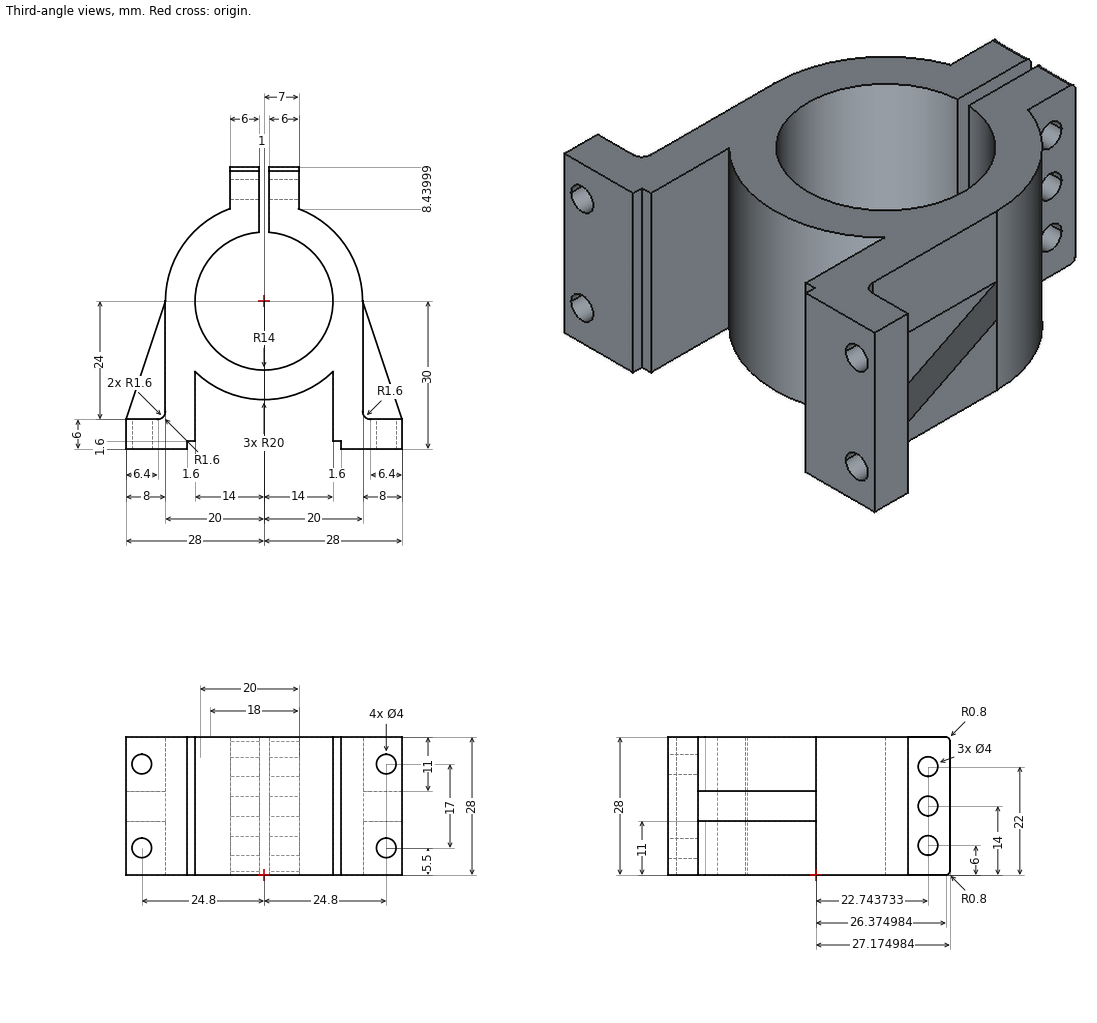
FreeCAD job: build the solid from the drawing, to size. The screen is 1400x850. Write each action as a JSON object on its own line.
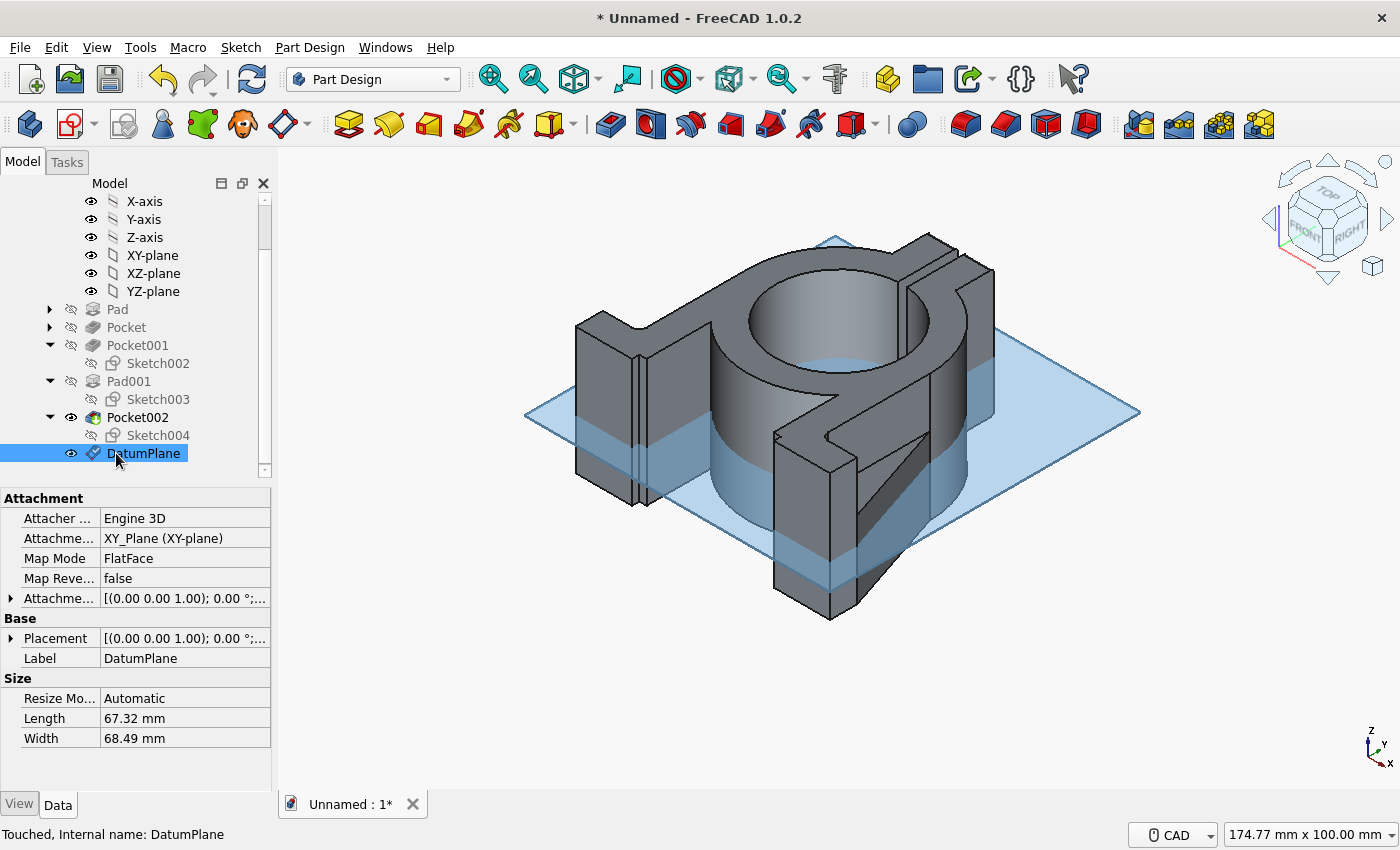
{"action": "left_click", "coordinate": [70, 124]}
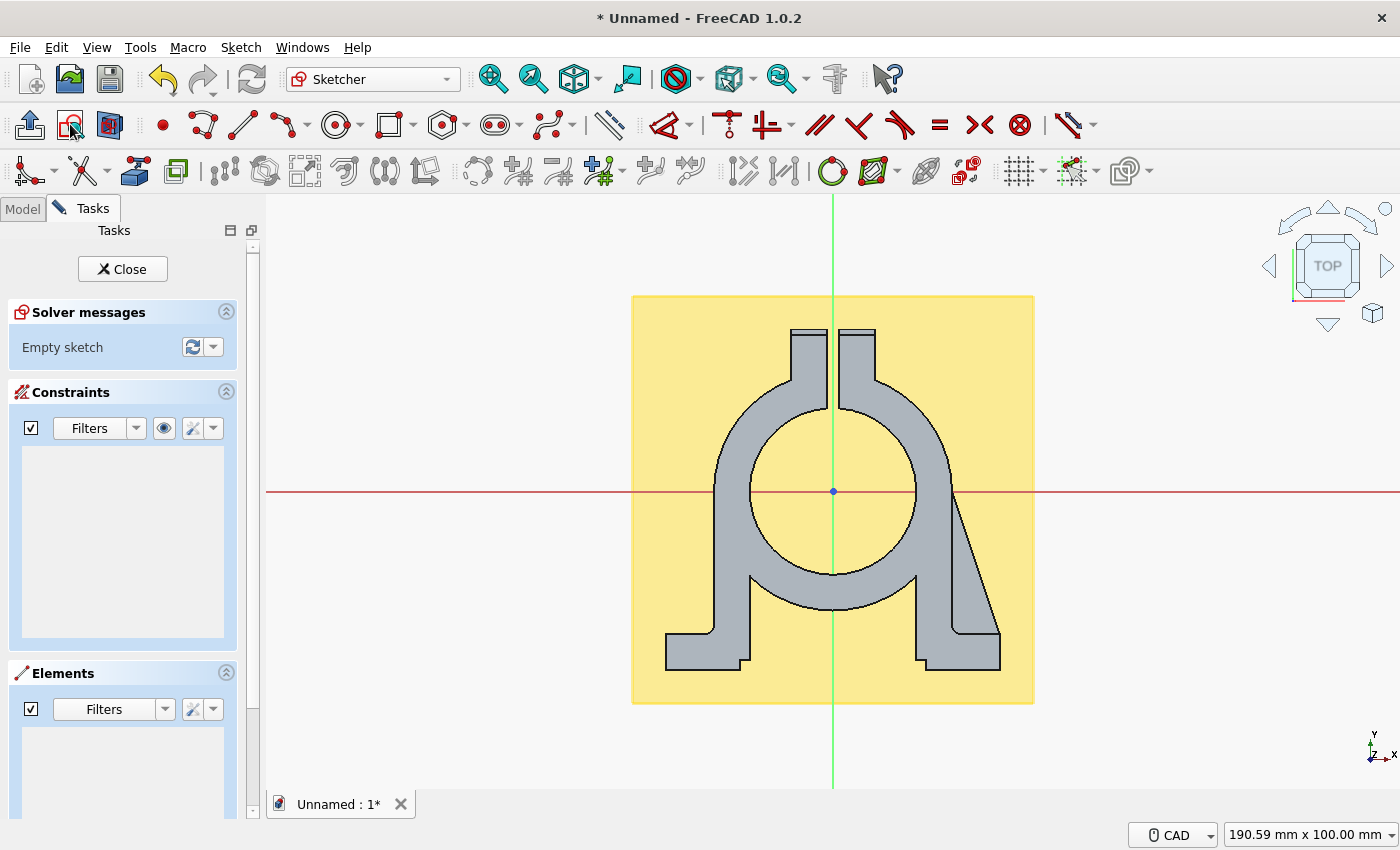
{"action": "left_click", "coordinate": [110, 126]}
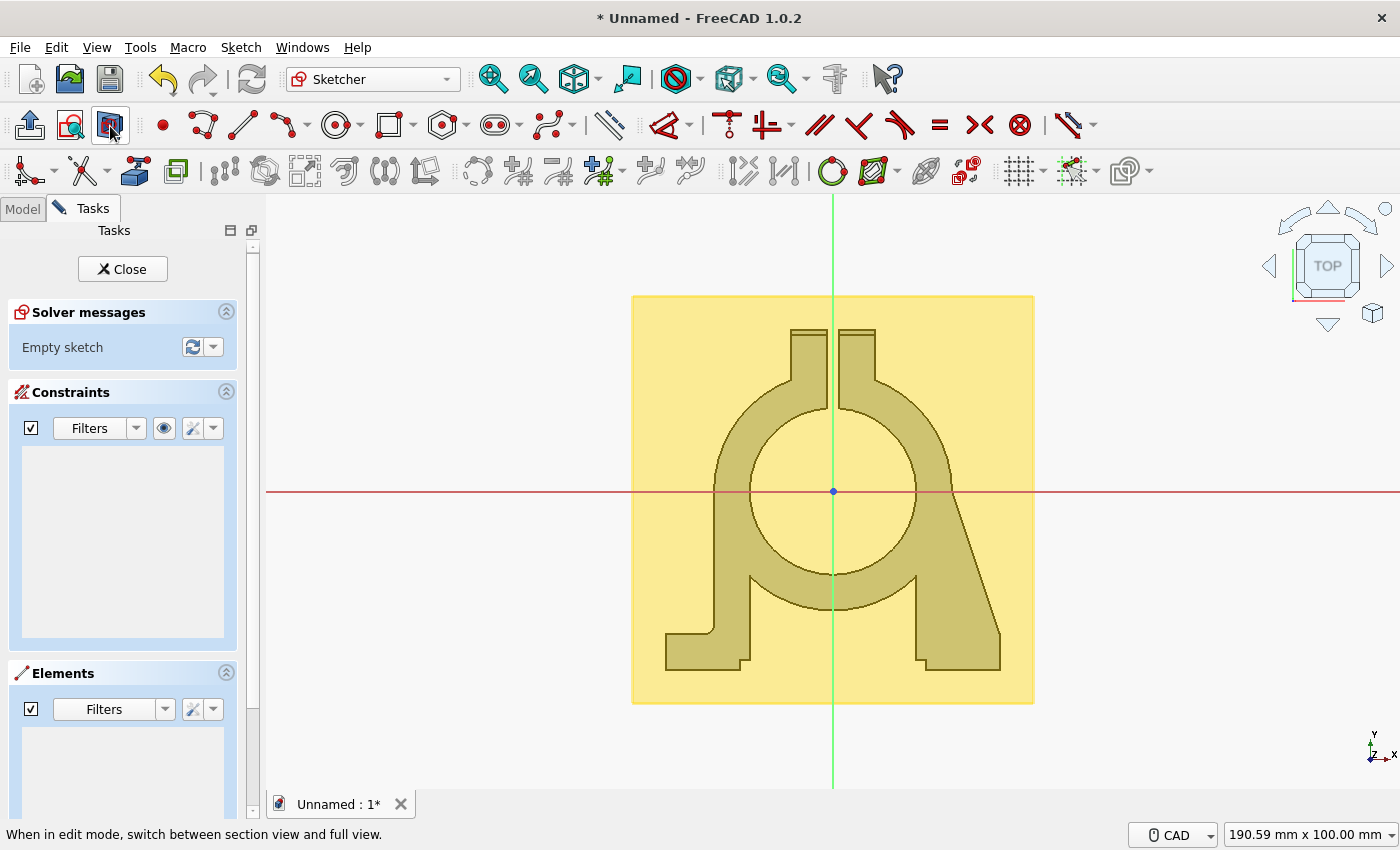
{"action": "scroll", "coordinate": [1005, 604], "scroll_direction": "up", "scroll_amount": 5}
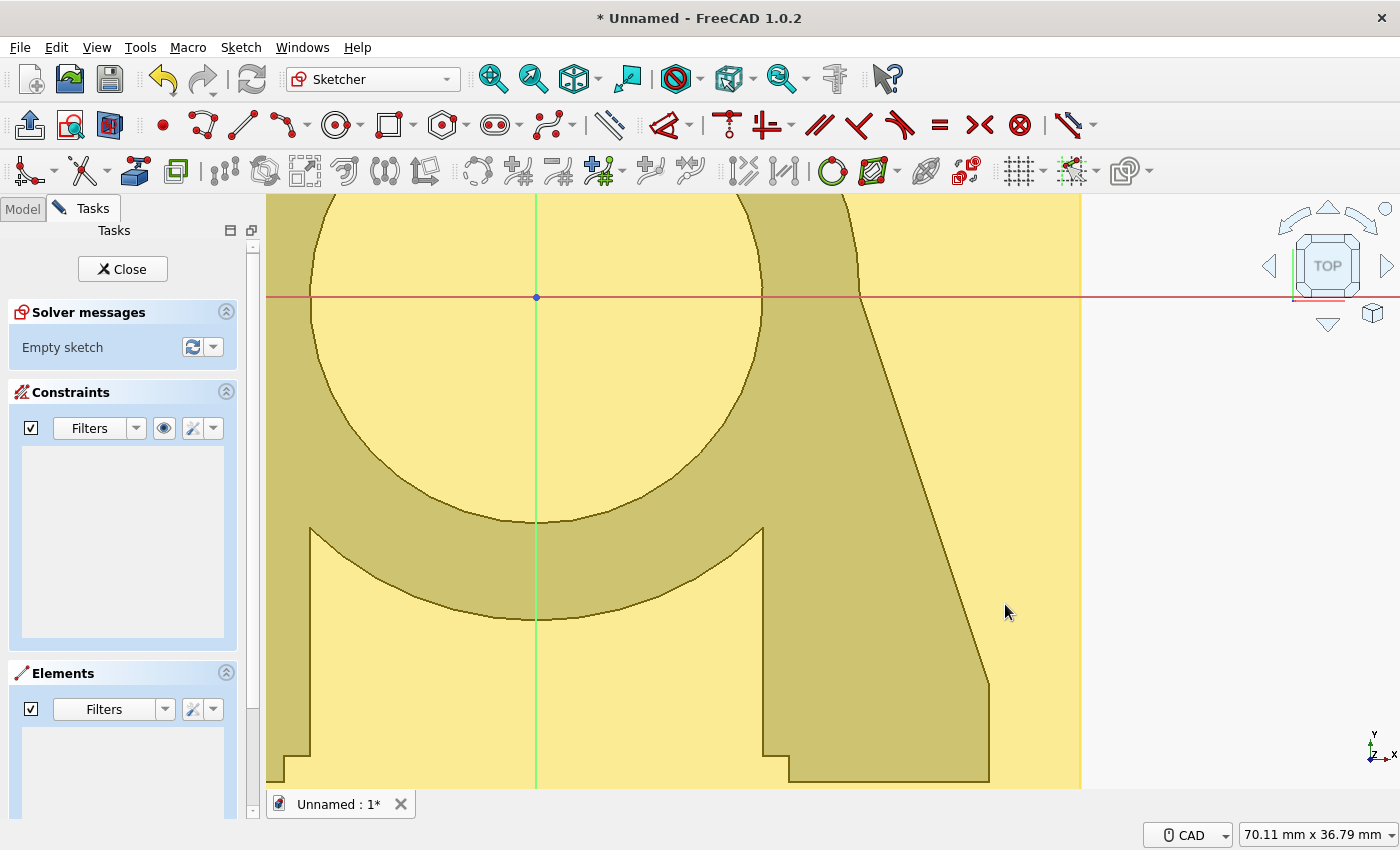
{"action": "left_click", "coordinate": [204, 126]}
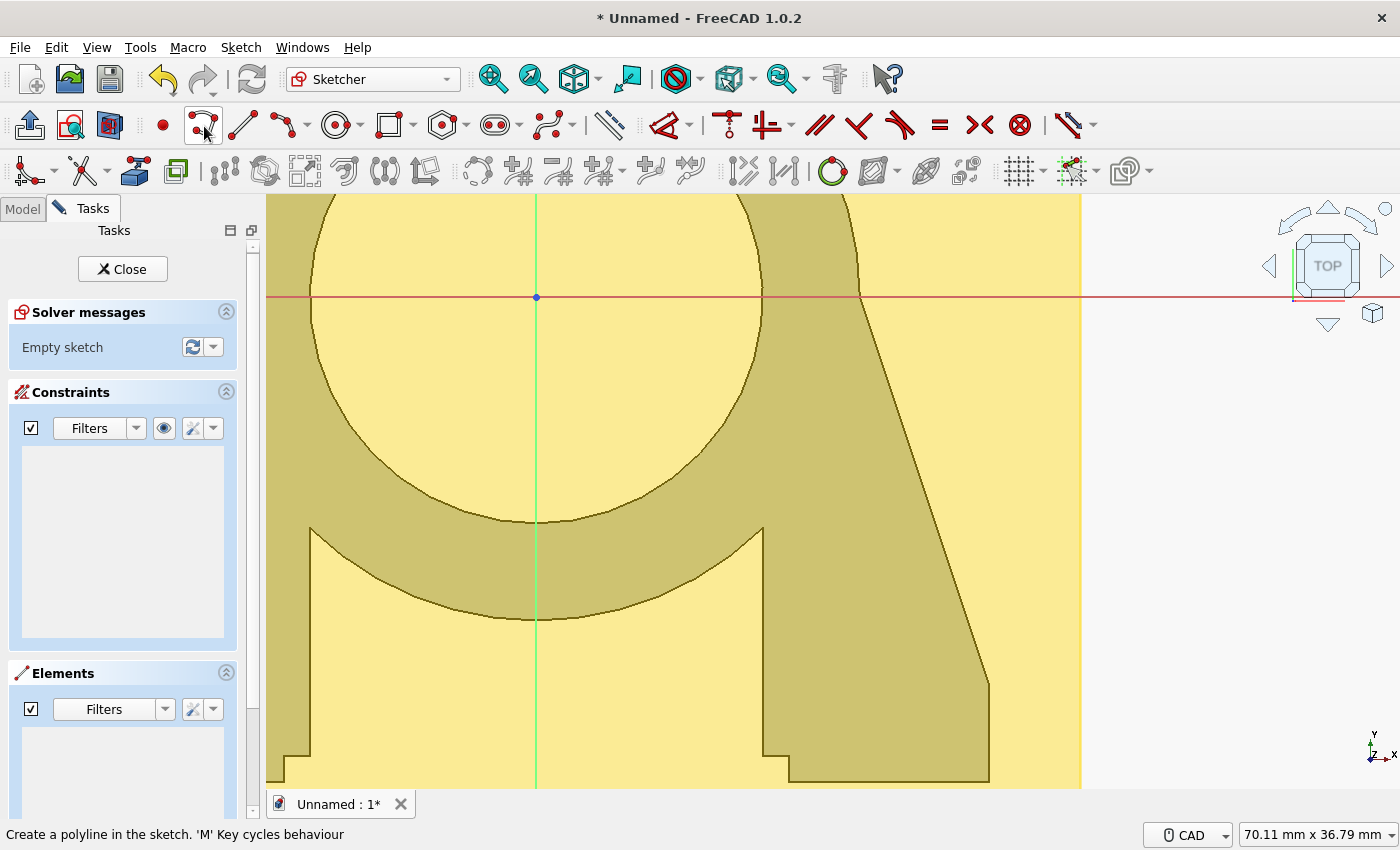
{"action": "left_click", "coordinate": [860, 659]}
{"action": "left_click", "coordinate": [860, 297]}
{"action": "left_click", "coordinate": [989, 685]}
{"action": "left_click", "coordinate": [886, 685]}
{"action": "right_click", "coordinate": [886, 685]}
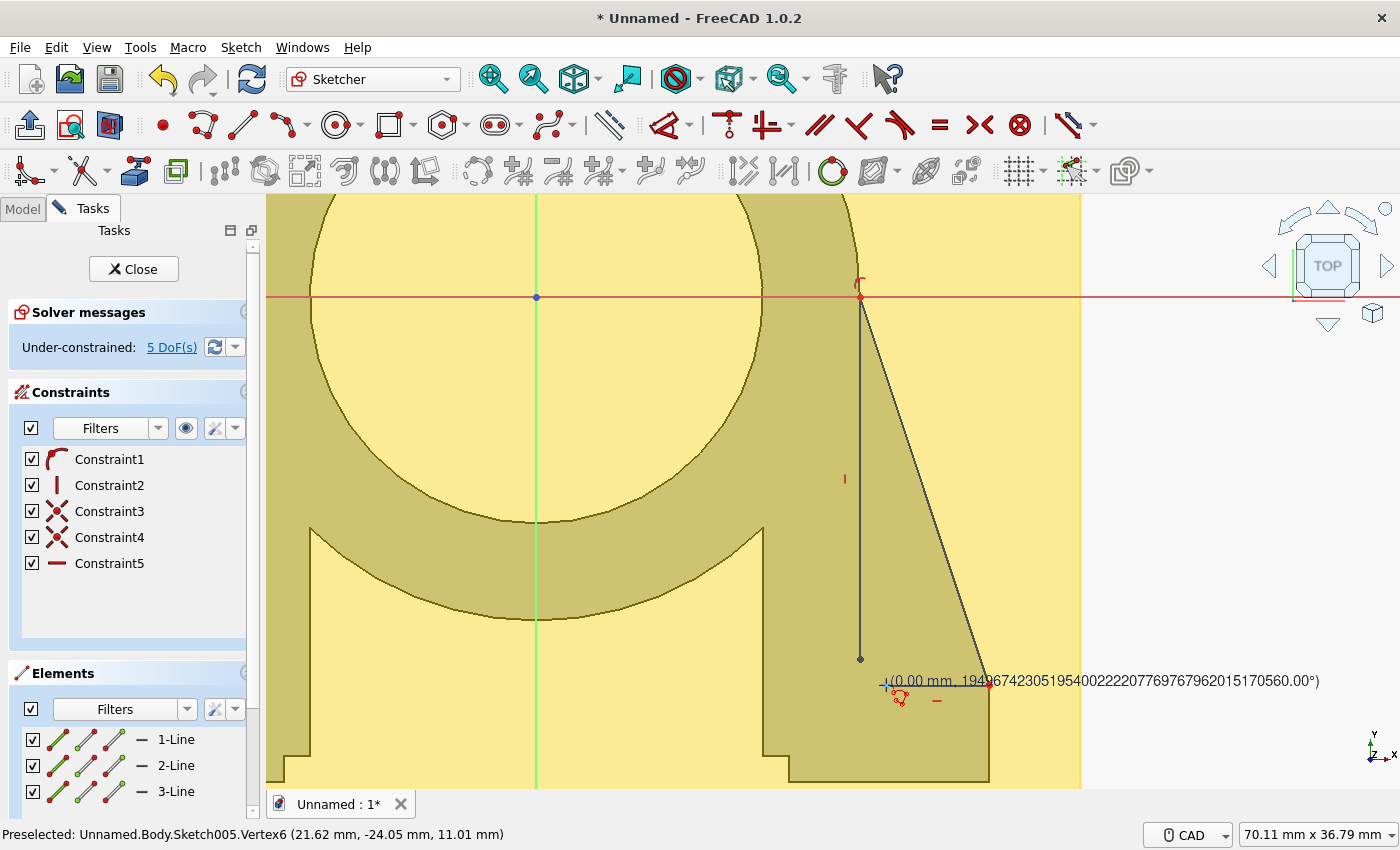
{"action": "left_click", "coordinate": [284, 126]}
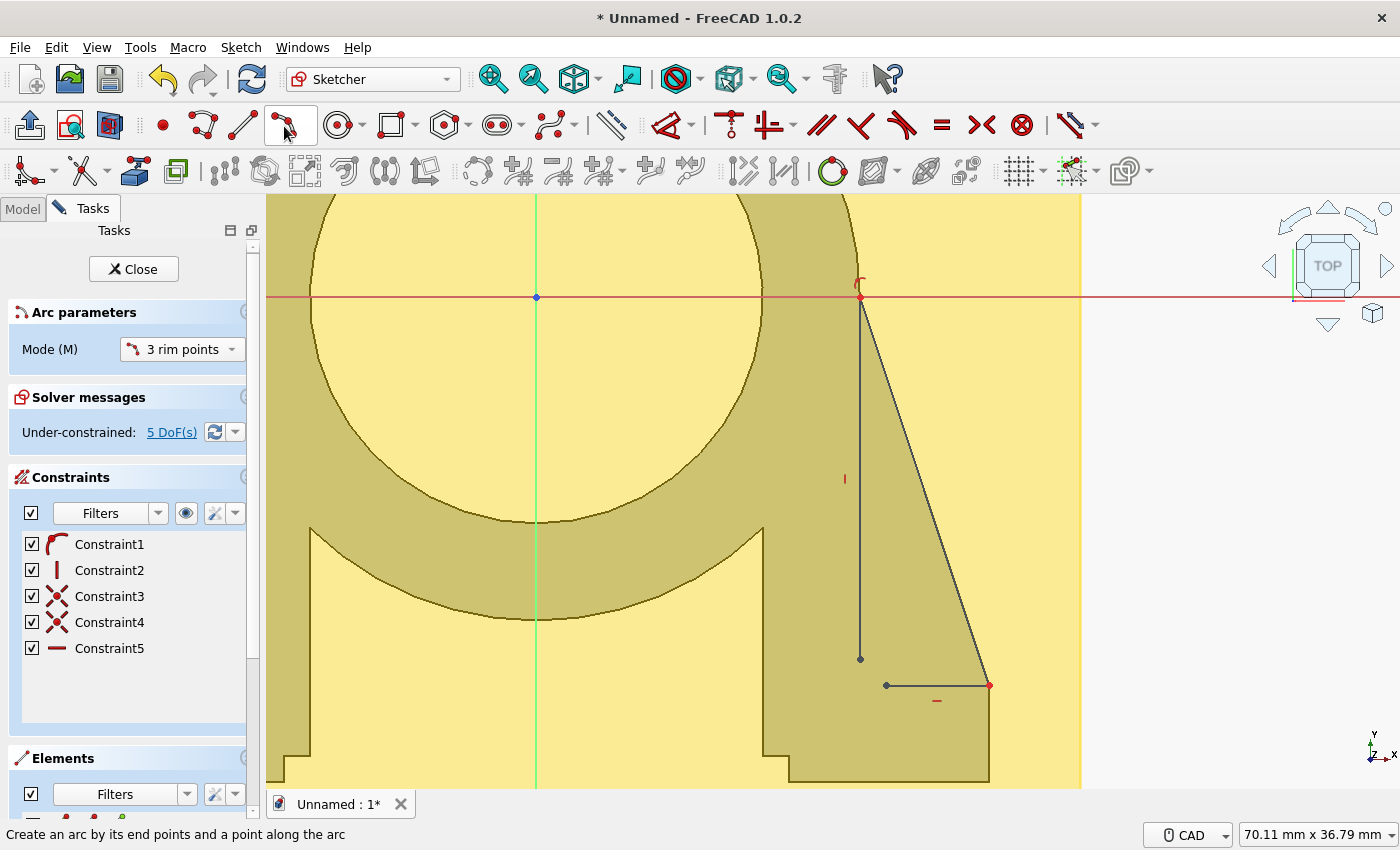
{"action": "left_click", "coordinate": [886, 686]}
{"action": "left_click", "coordinate": [860, 660]}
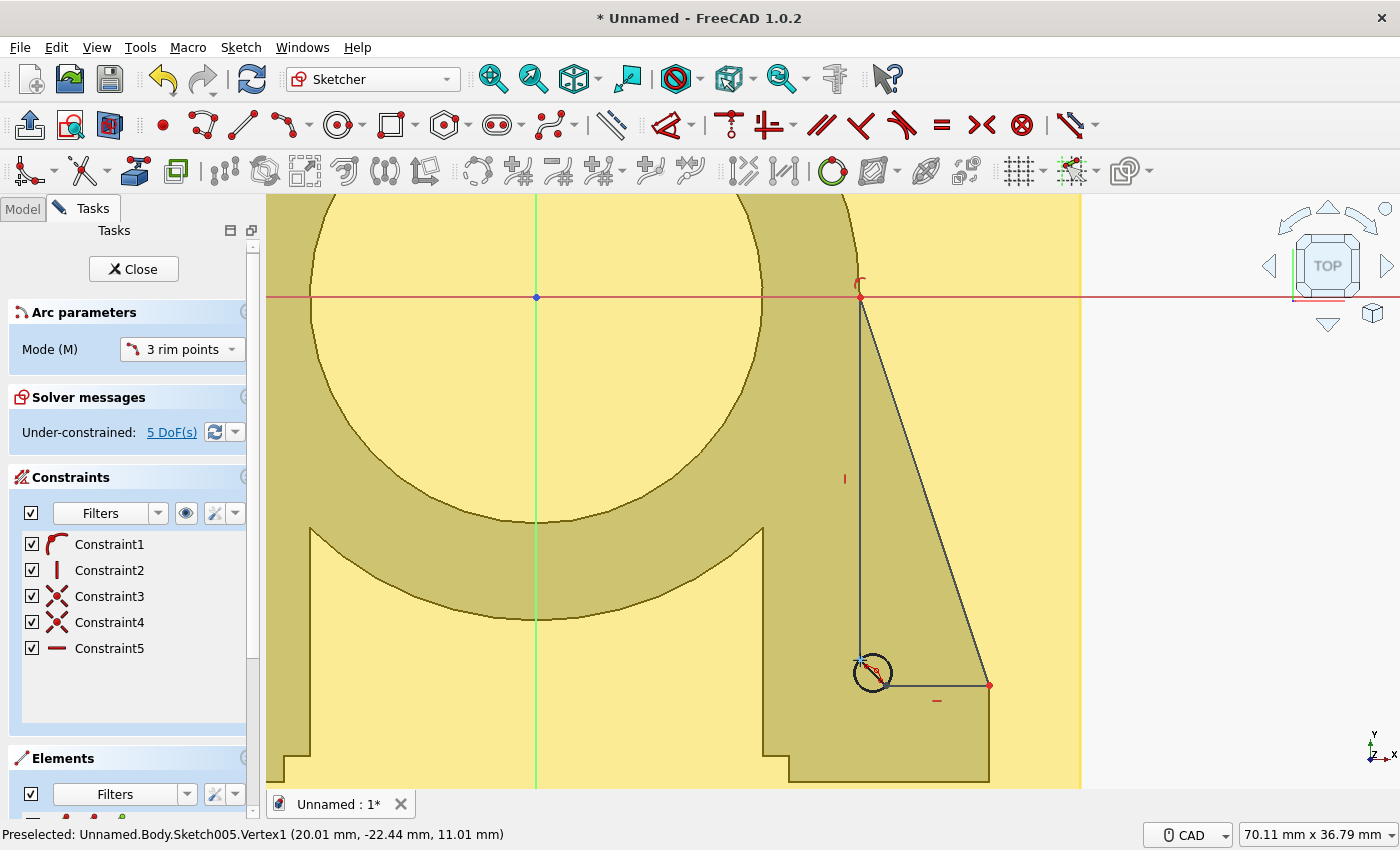
{"action": "scroll", "coordinate": [867, 678], "scroll_direction": "up", "scroll_amount": 4}